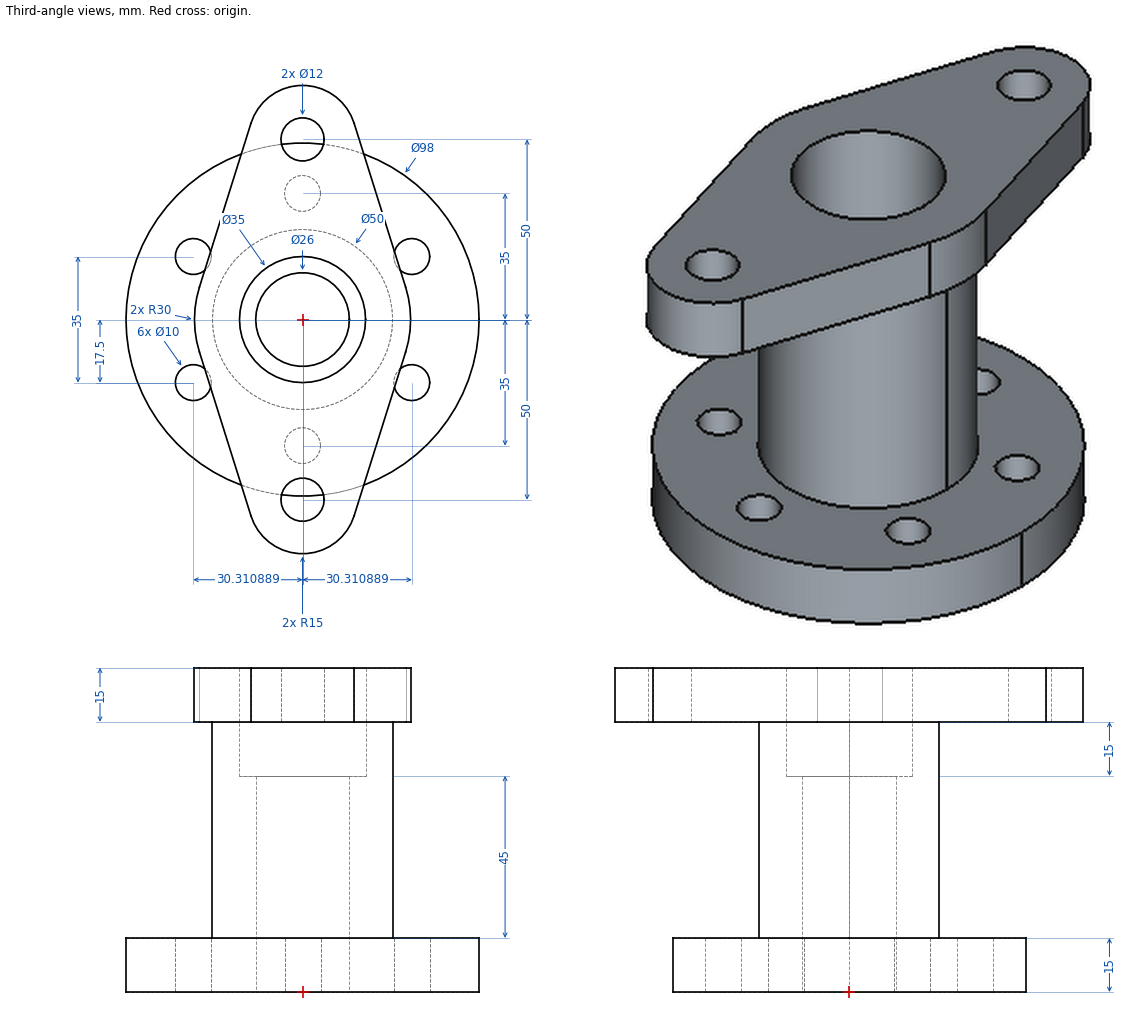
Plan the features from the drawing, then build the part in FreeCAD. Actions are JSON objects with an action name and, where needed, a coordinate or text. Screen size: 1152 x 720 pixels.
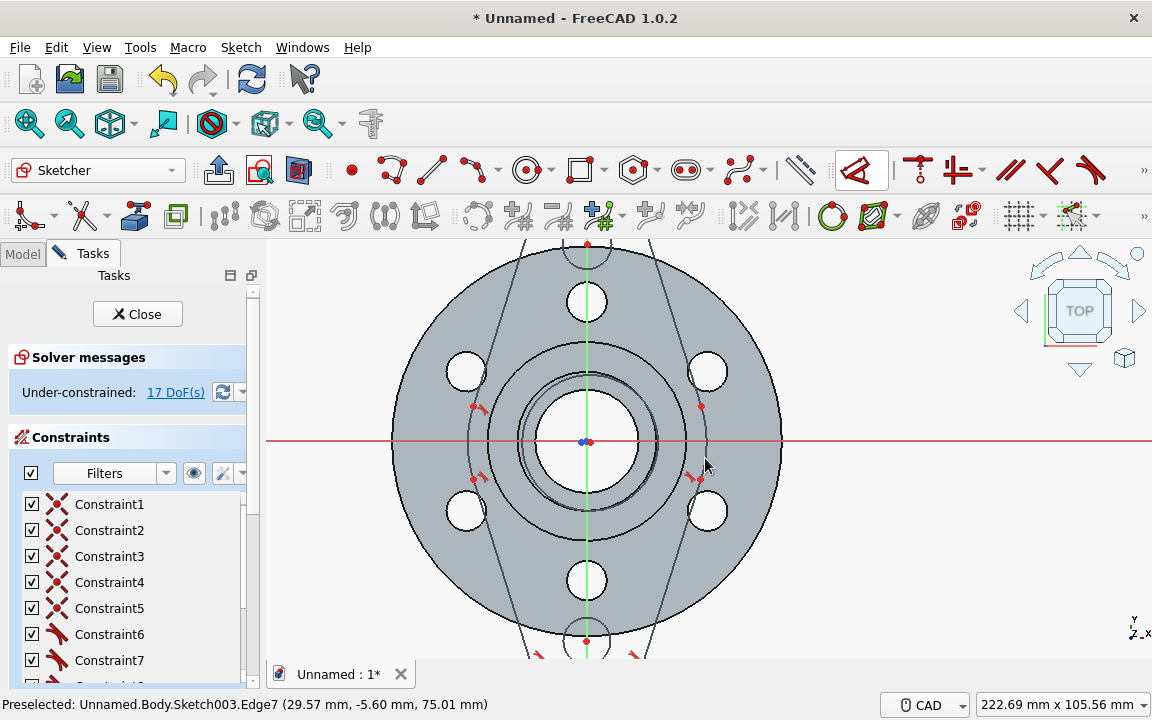
{"action": "left_click", "coordinate": [684, 352]}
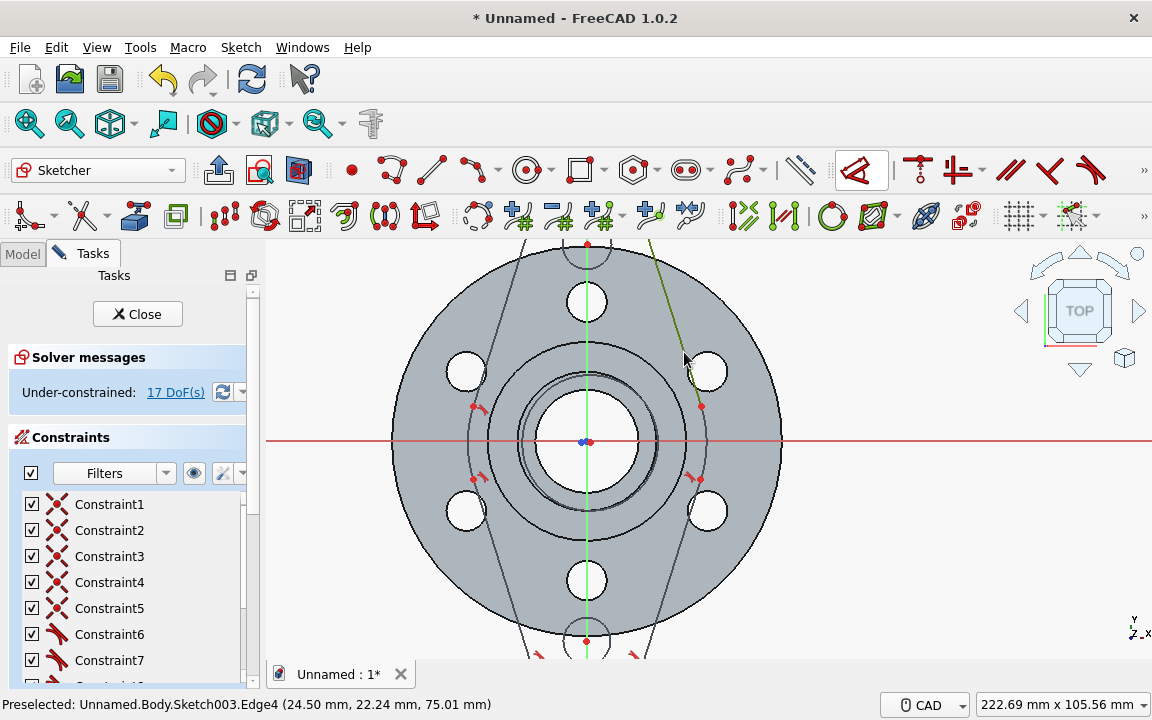
{"action": "left_click", "coordinate": [706, 458]}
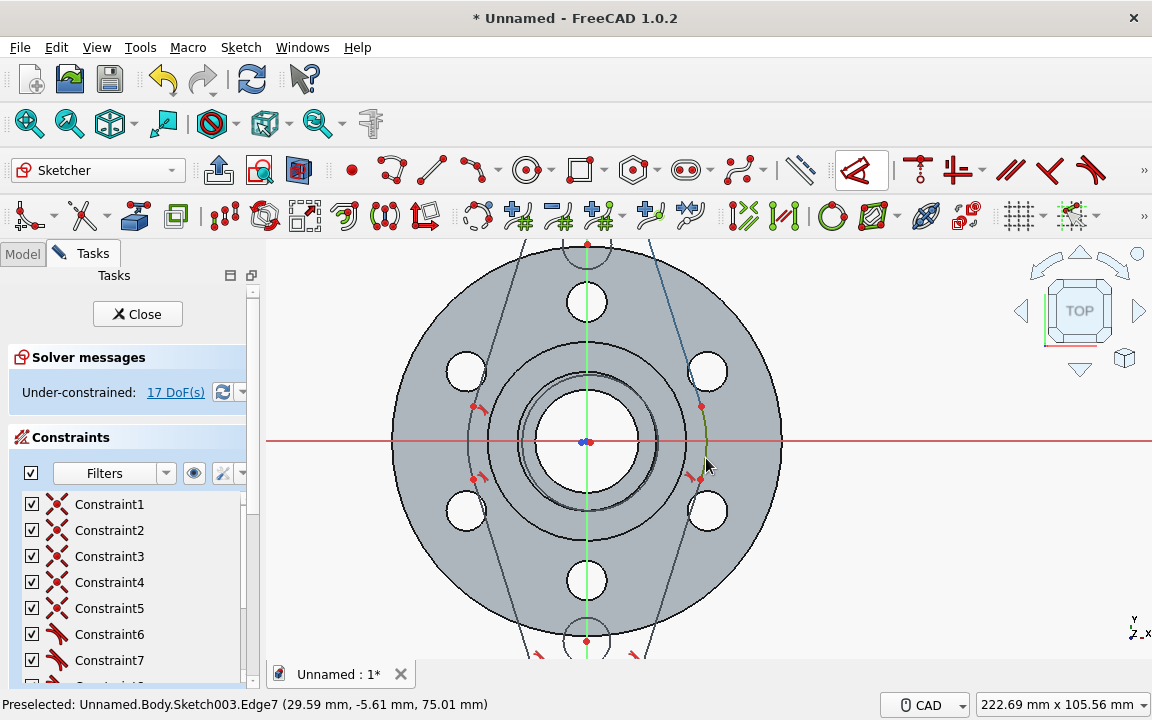
{"action": "key", "text": "t"}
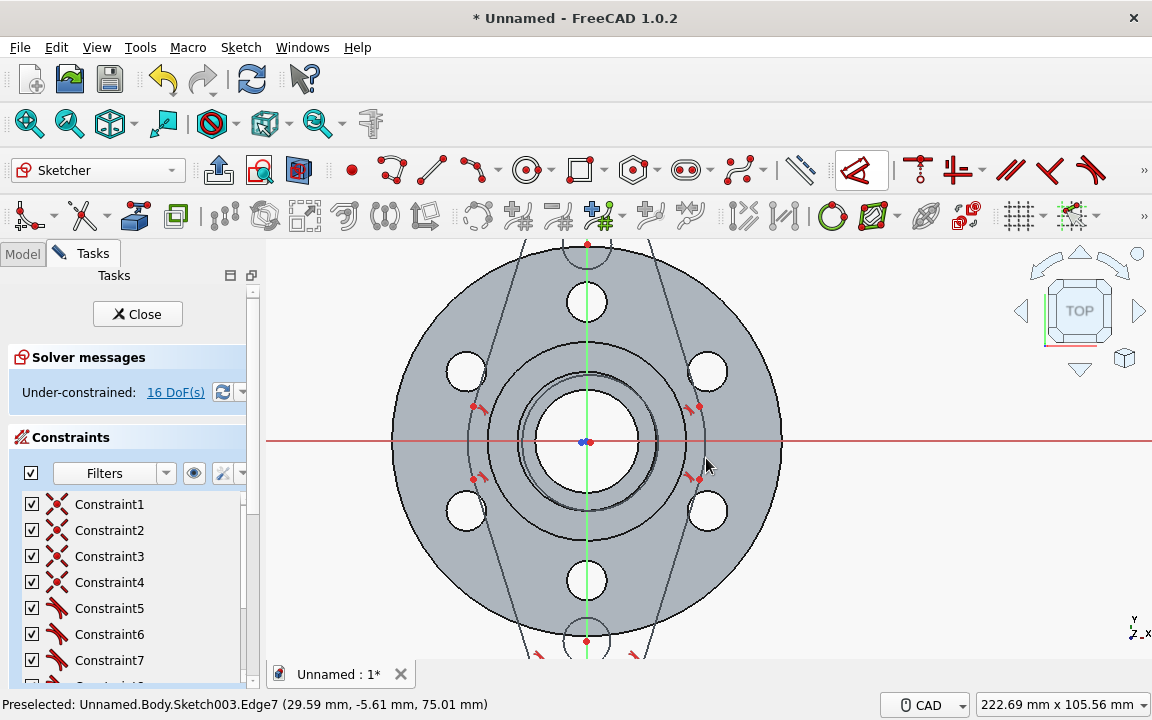
{"action": "left_click", "coordinate": [683, 352]}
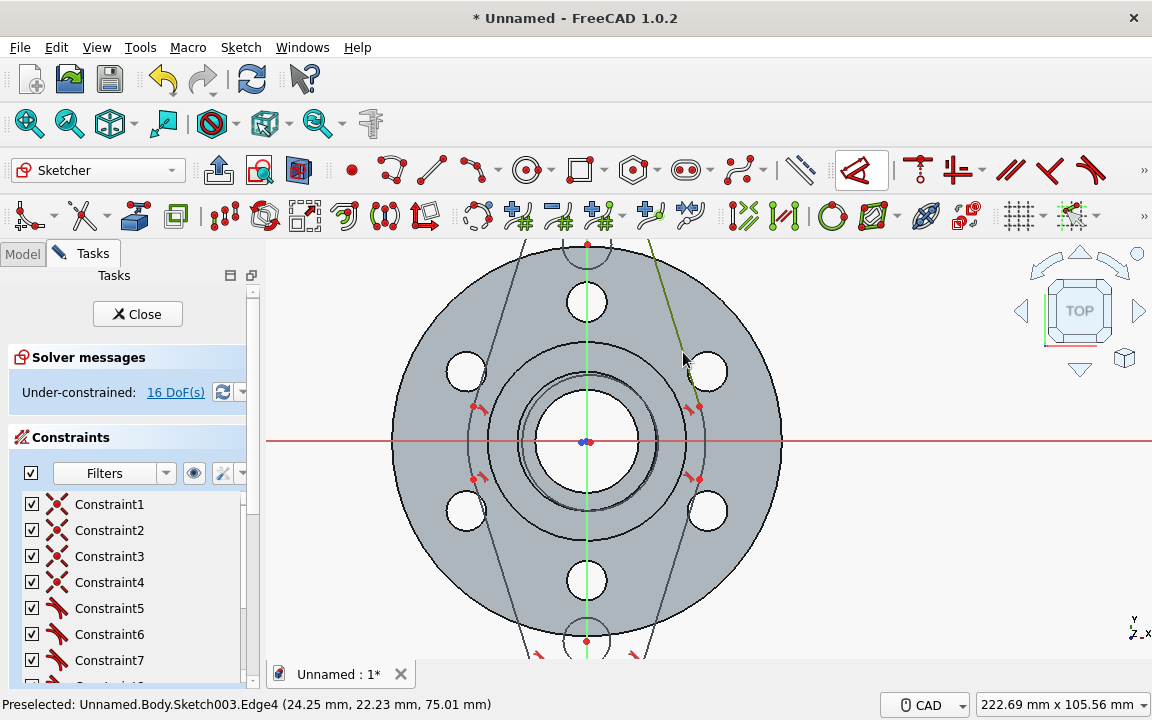
{"action": "scroll", "coordinate": [706, 458], "scroll_direction": "down", "scroll_amount": 3}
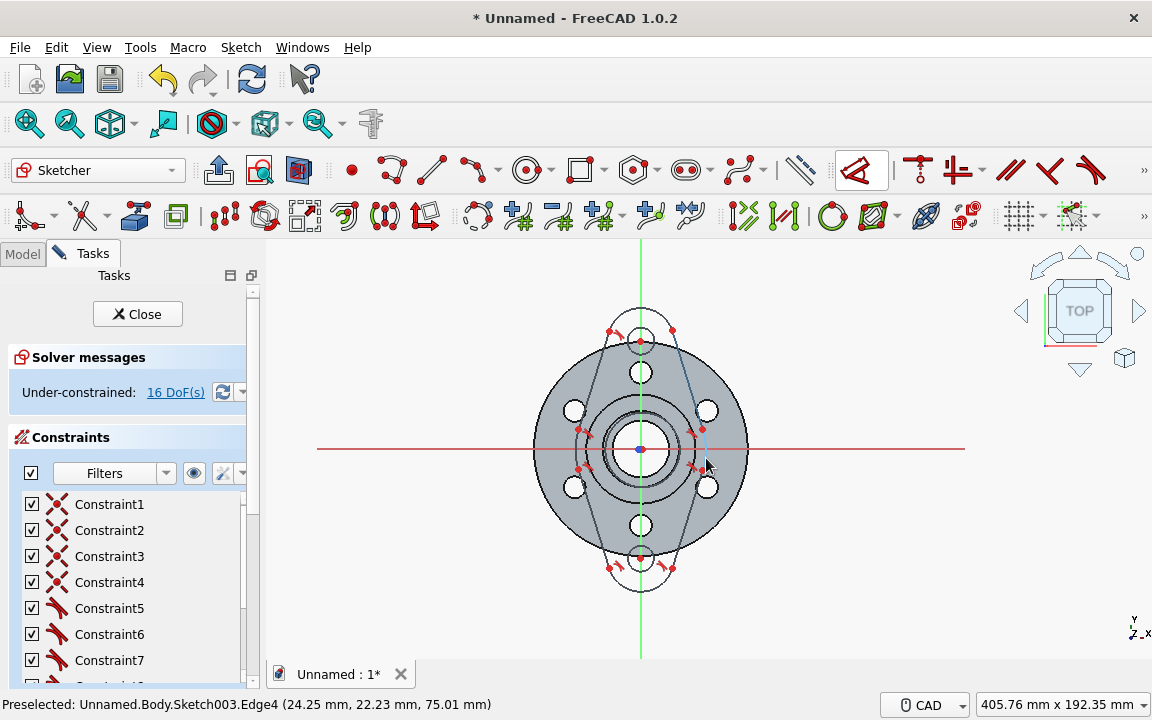
{"action": "left_click", "coordinate": [657, 312]}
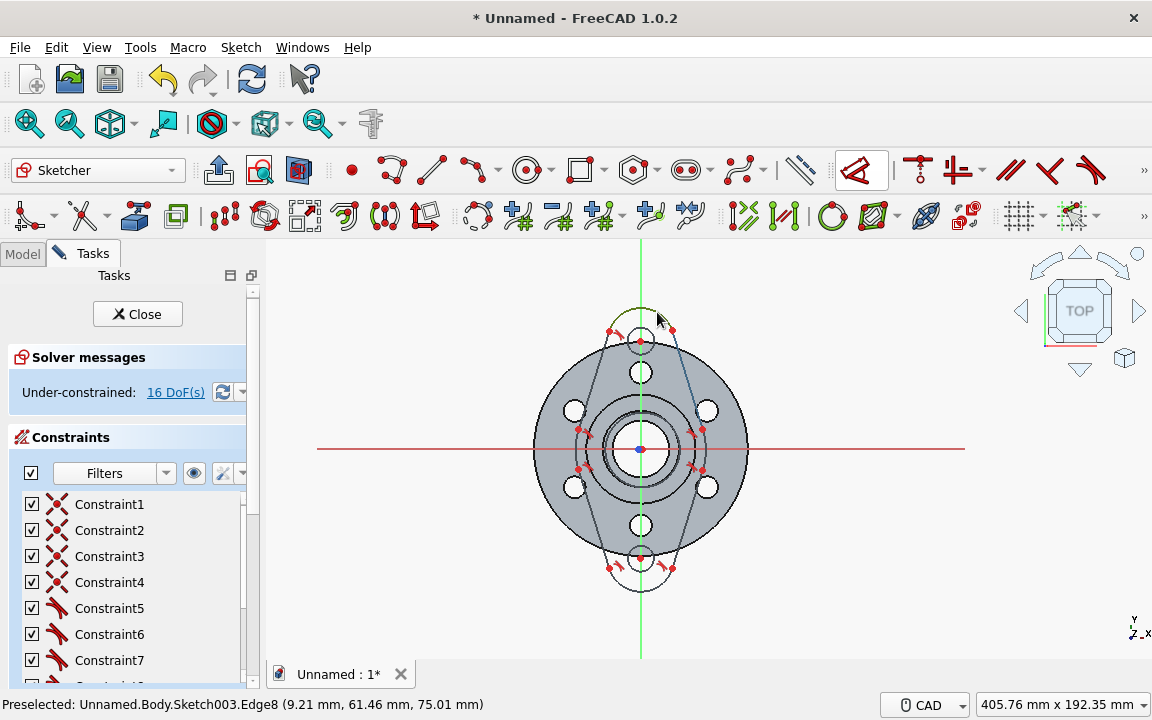
{"action": "left_click", "coordinate": [1092, 170]}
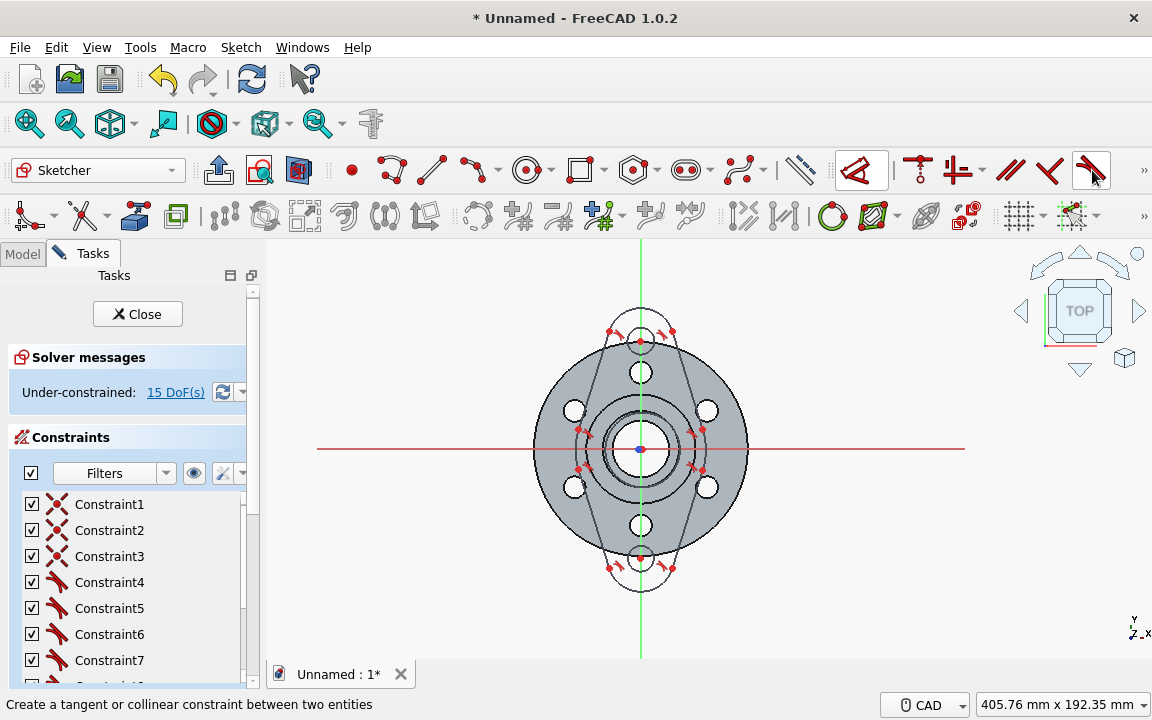
{"action": "left_click", "coordinate": [669, 424]}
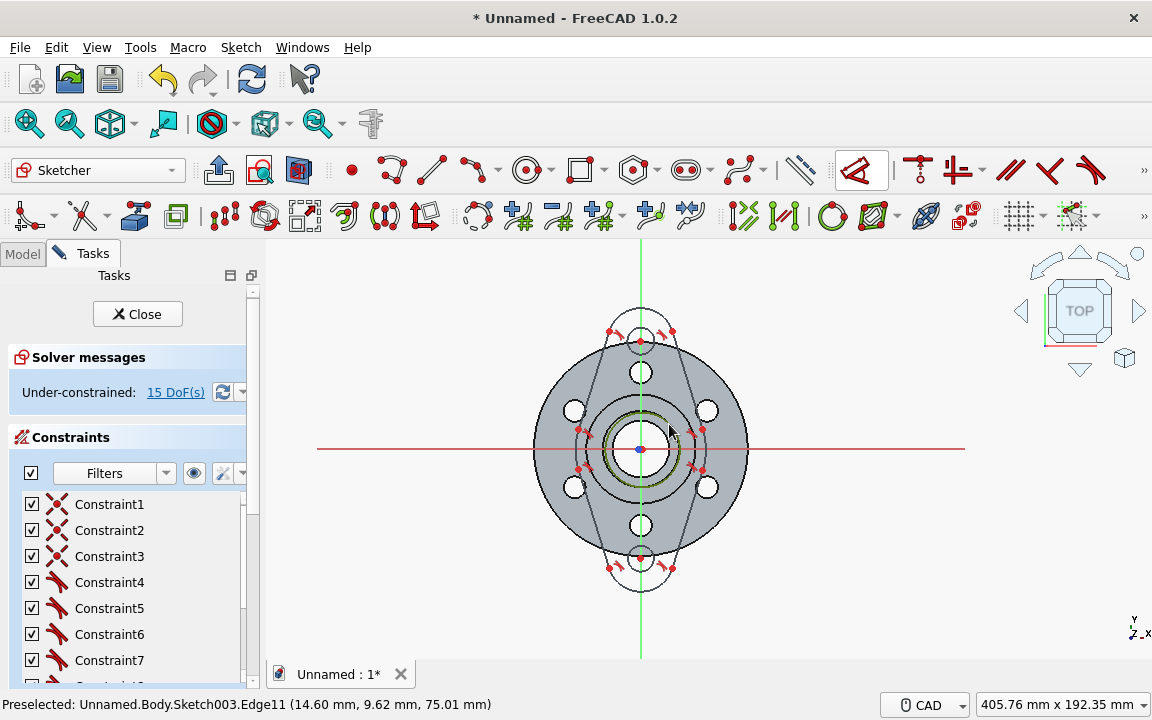
{"action": "scroll", "coordinate": [705, 458], "scroll_direction": "up", "scroll_amount": 3}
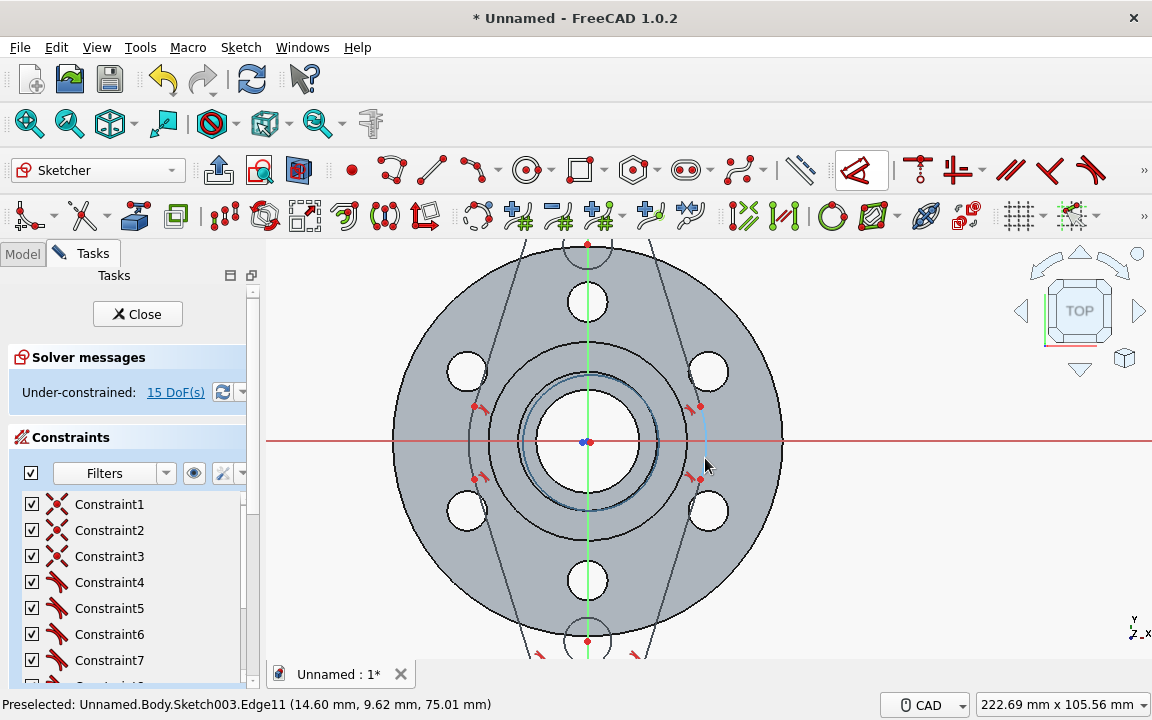
{"action": "left_click", "coordinate": [705, 458]}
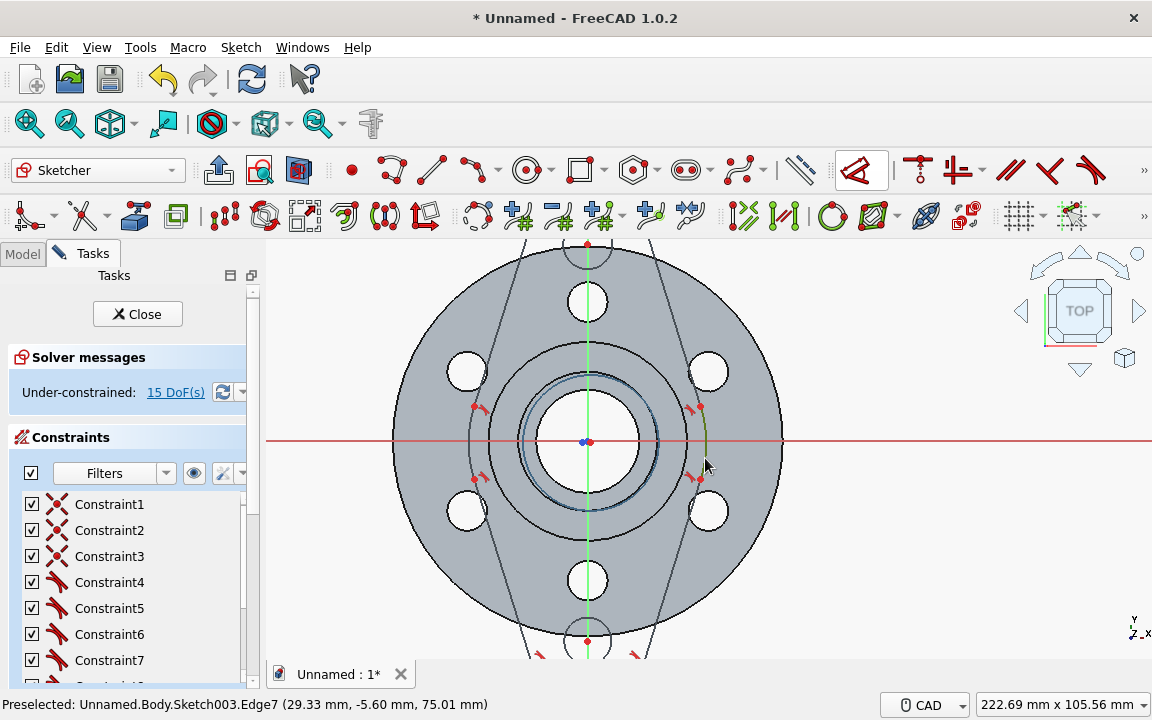
{"action": "key", "text": "c"}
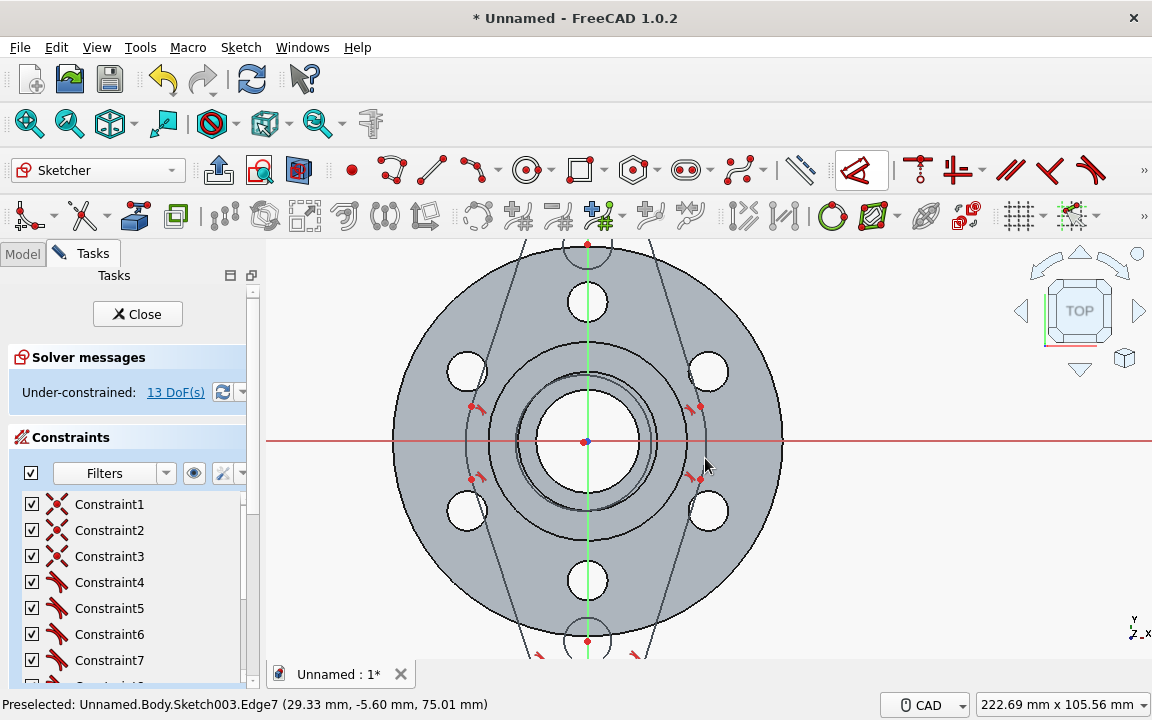
{"action": "scroll", "coordinate": [586, 442], "scroll_direction": "up", "scroll_amount": 3}